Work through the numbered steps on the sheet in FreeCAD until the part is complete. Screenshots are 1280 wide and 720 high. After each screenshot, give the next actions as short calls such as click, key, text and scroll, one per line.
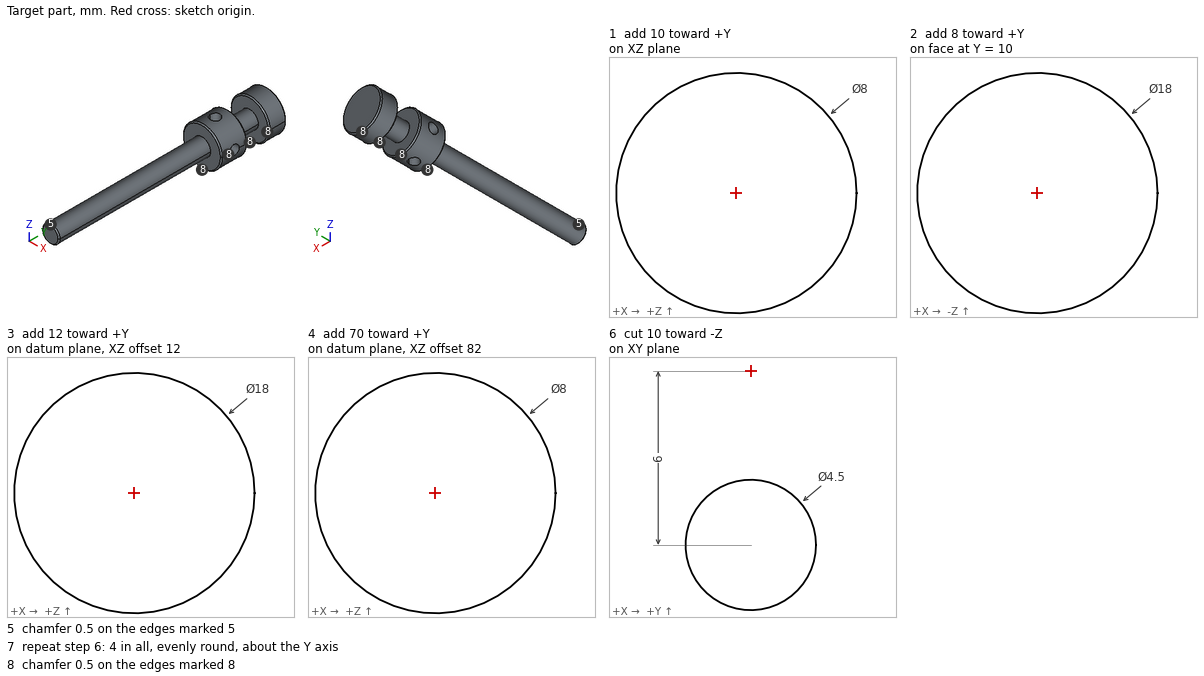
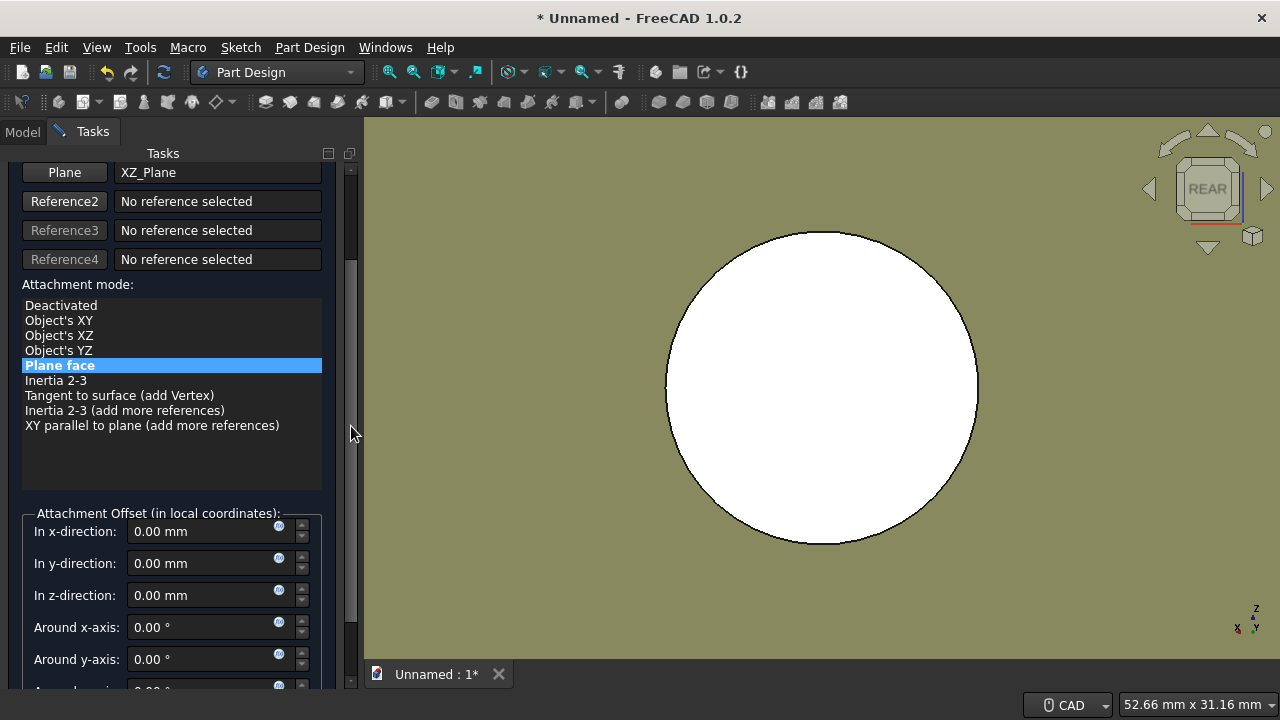
triple_click(210, 595)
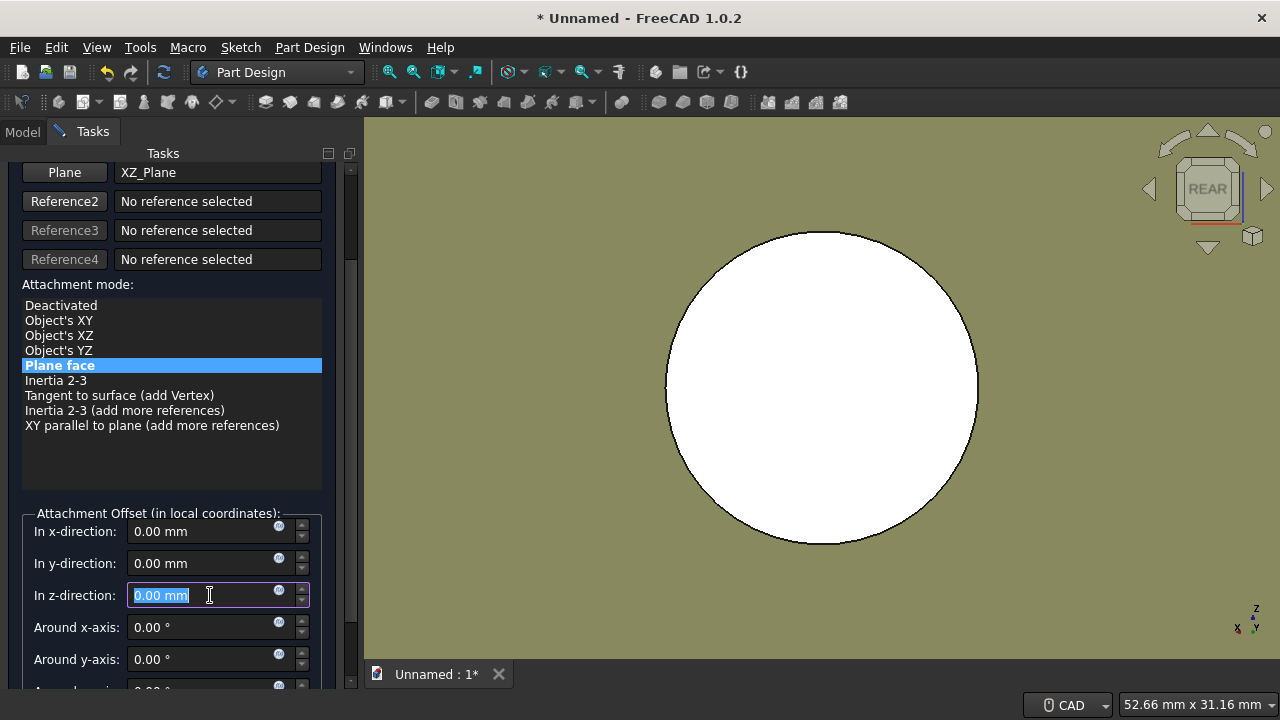
text(82)
key(Tab)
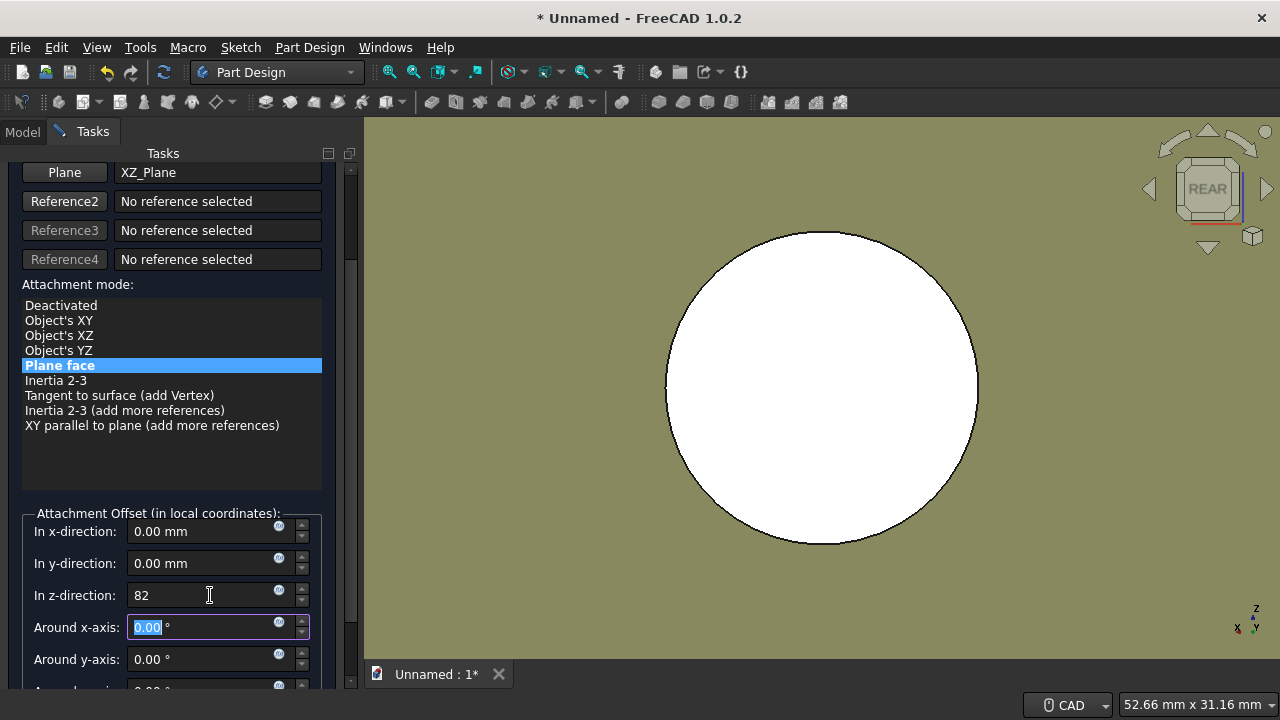
scroll(351, 426, up, 3)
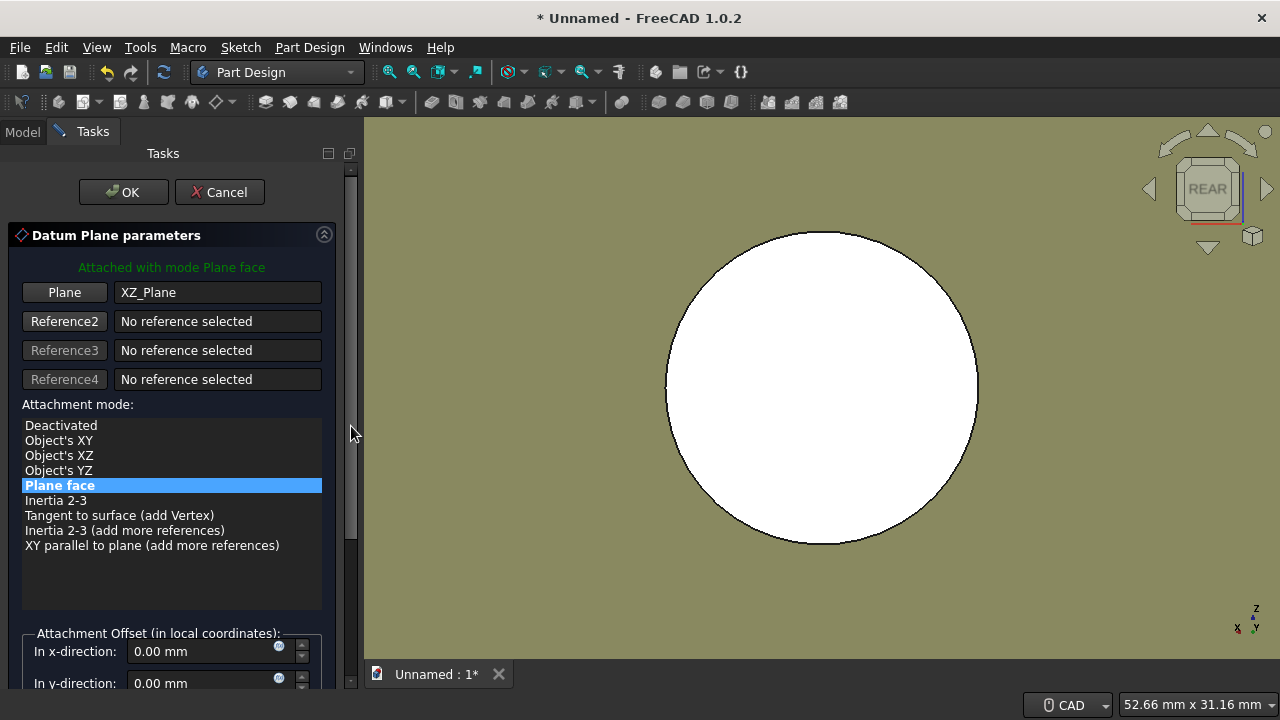
click(124, 192)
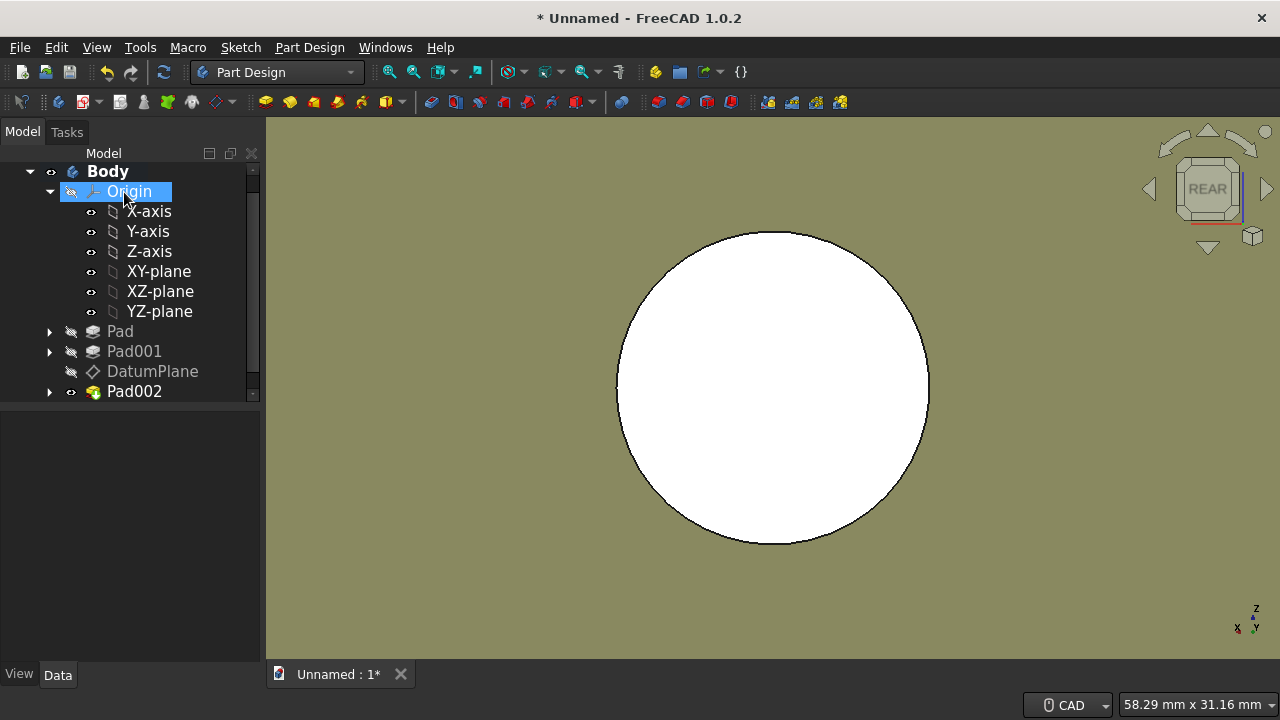
scroll(120, 287, down, 3)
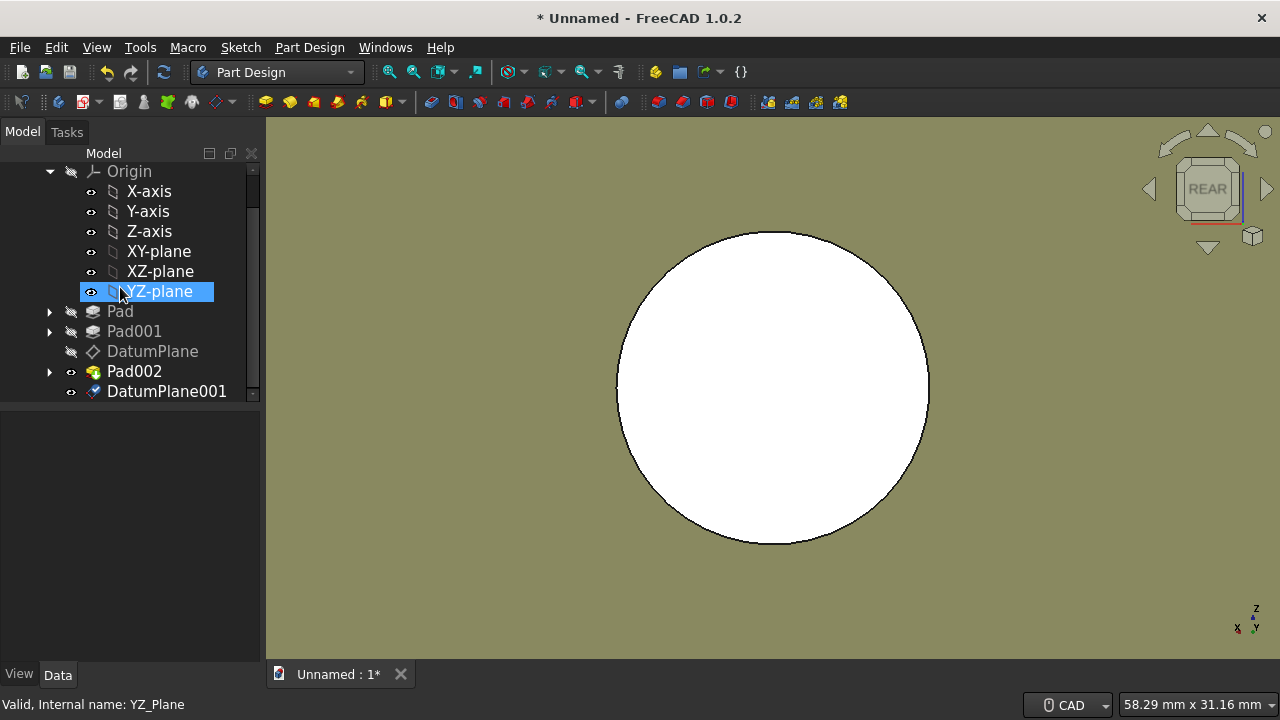
click(116, 392)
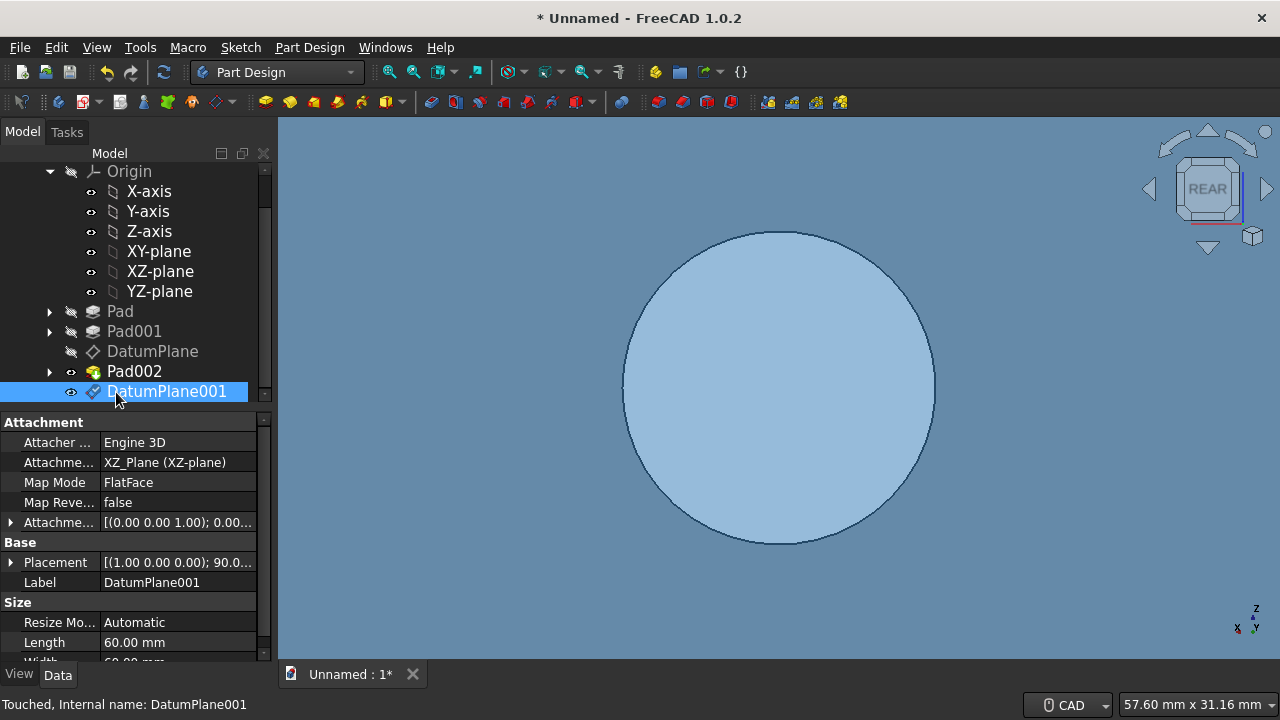
click(84, 102)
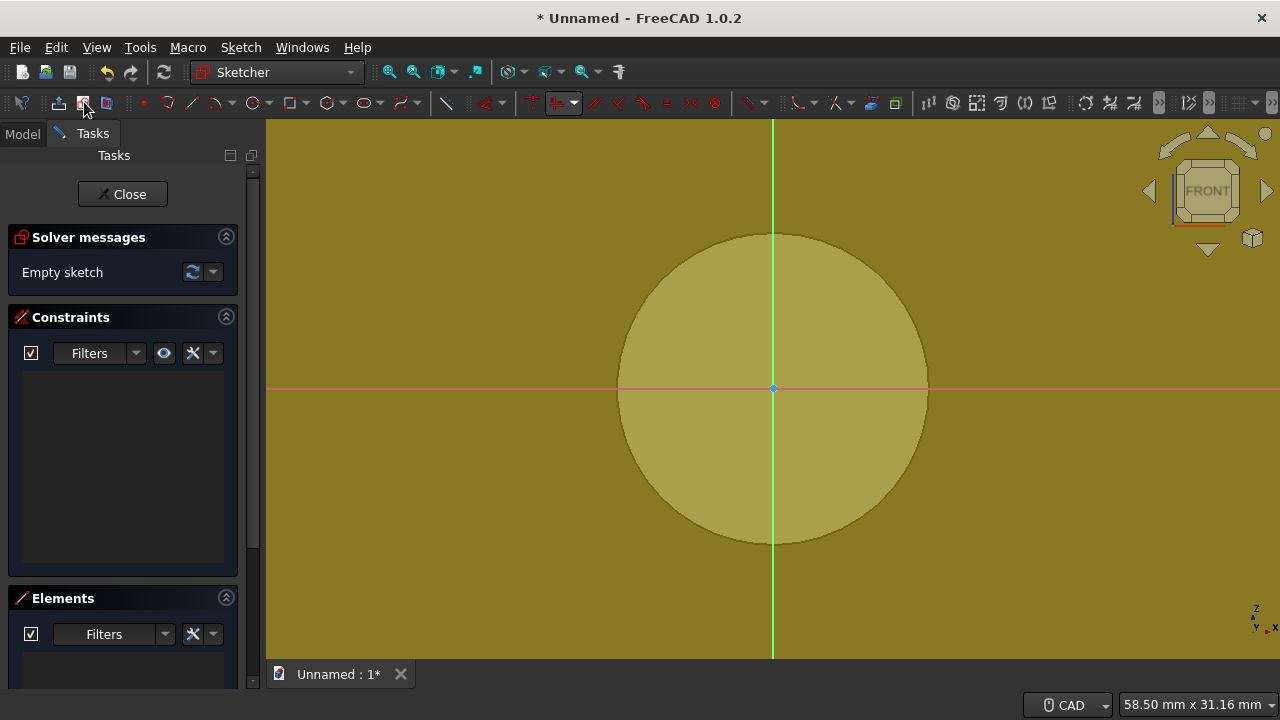
scroll(813, 389, up, 5)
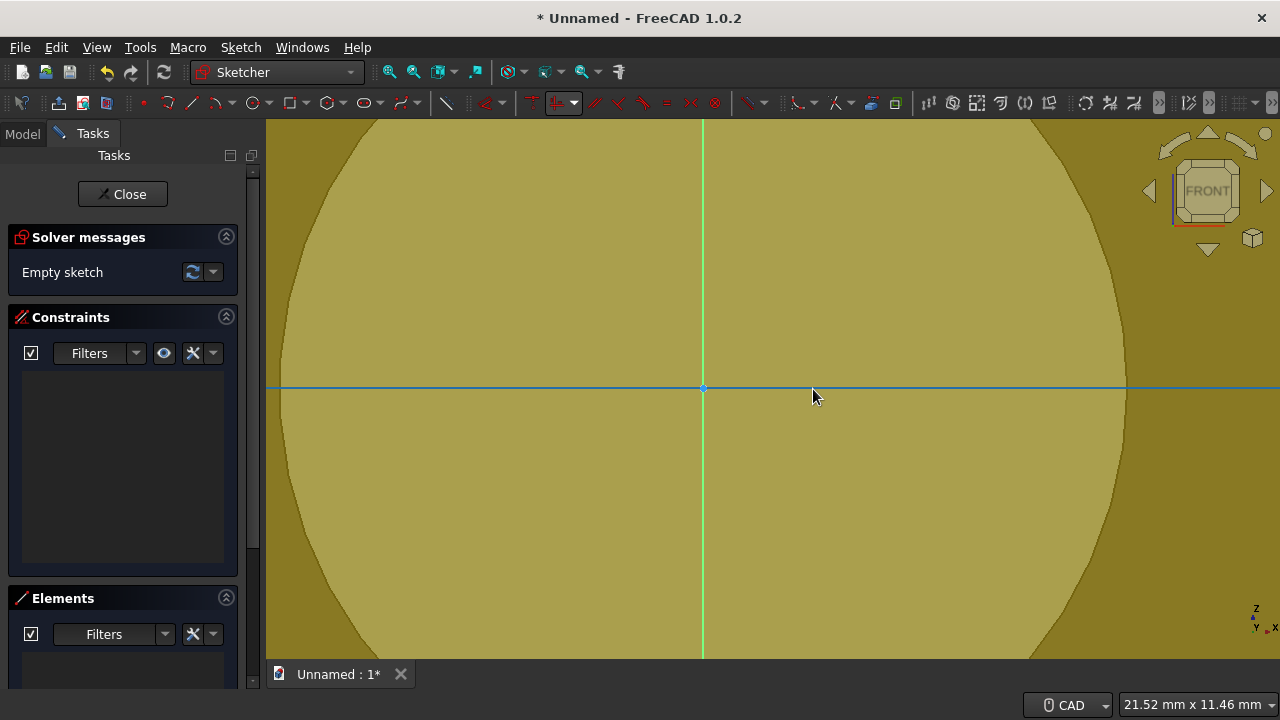
click(254, 104)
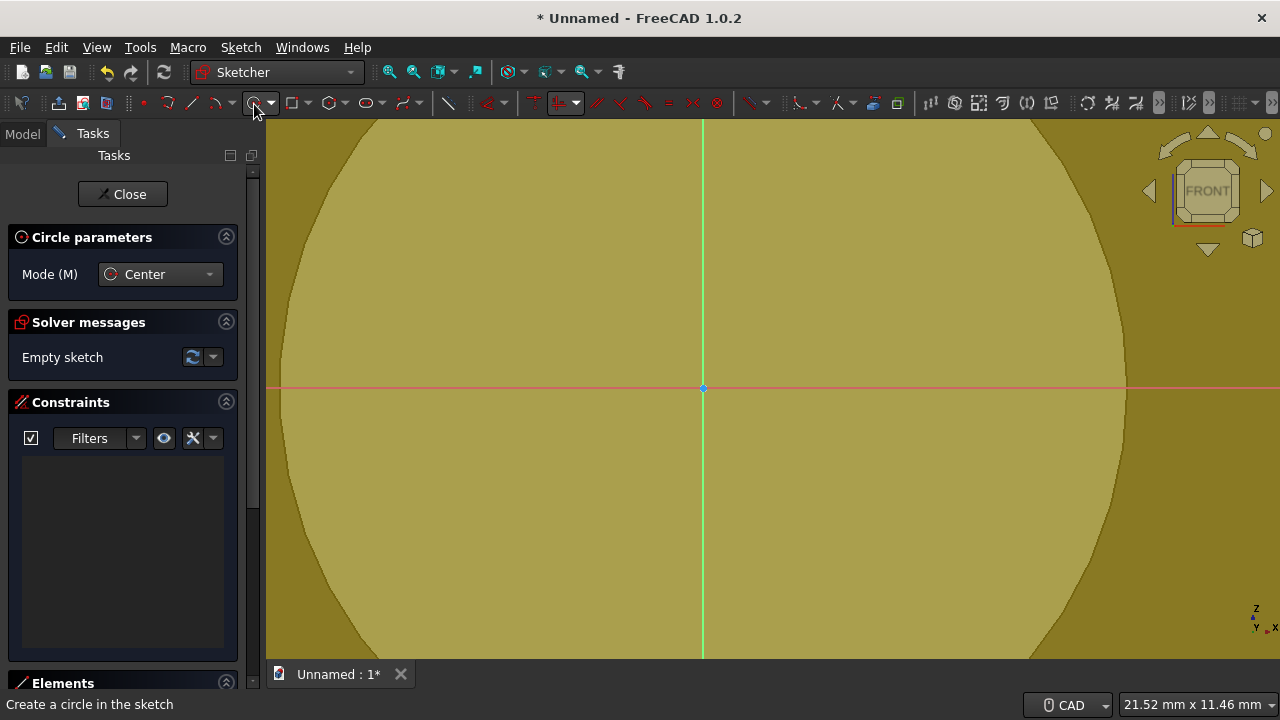
click(703, 388)
click(837, 255)
key(Escape)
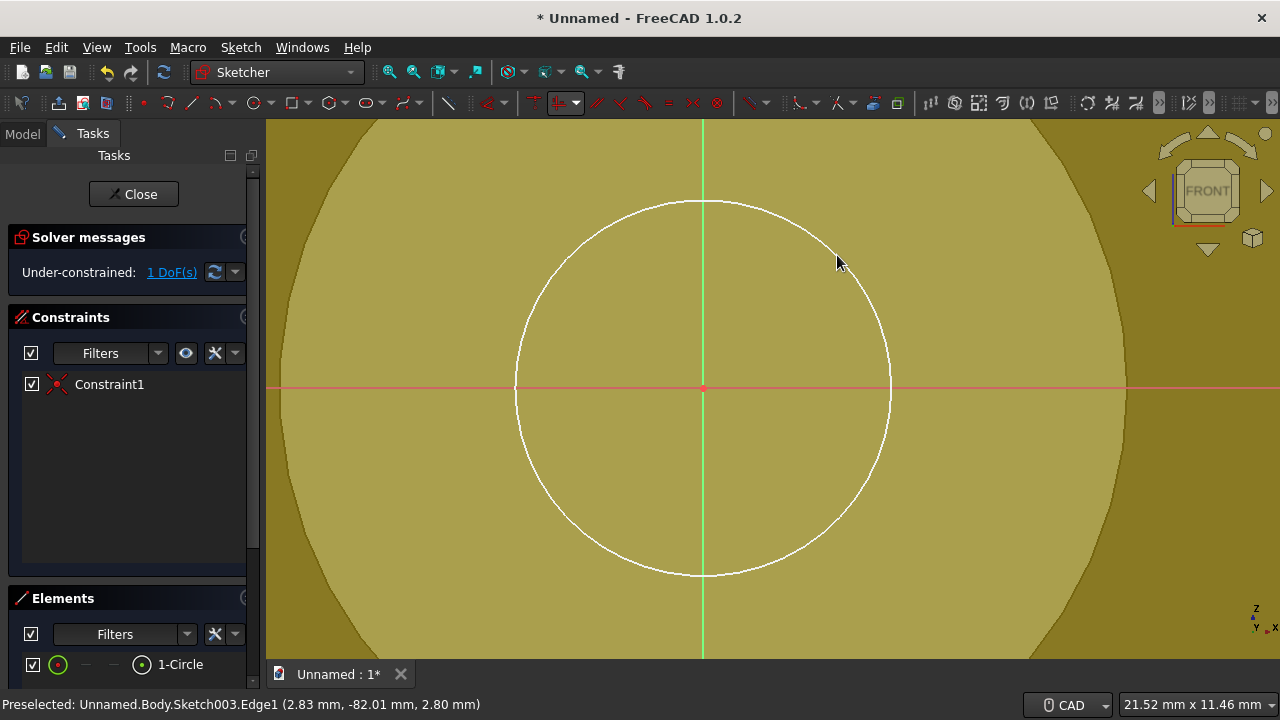
click(488, 104)